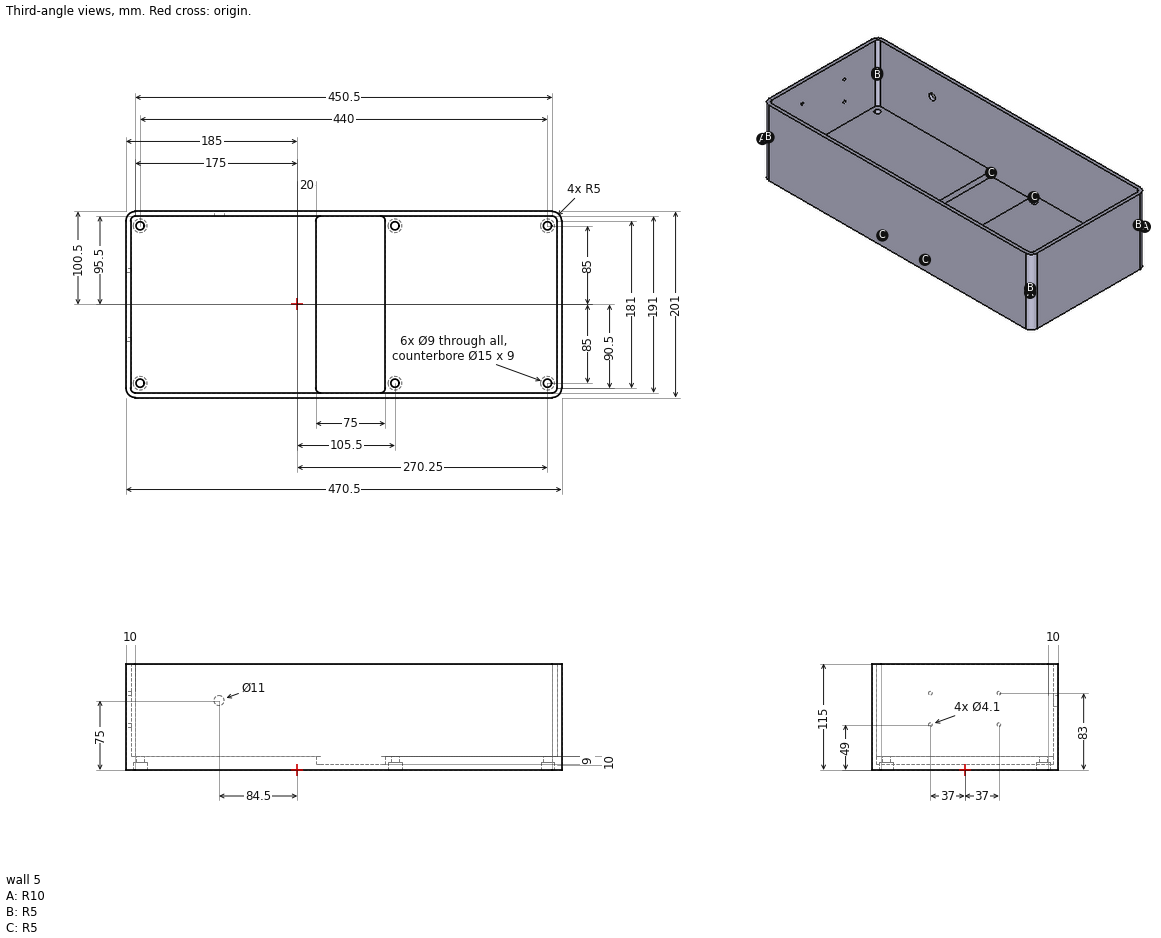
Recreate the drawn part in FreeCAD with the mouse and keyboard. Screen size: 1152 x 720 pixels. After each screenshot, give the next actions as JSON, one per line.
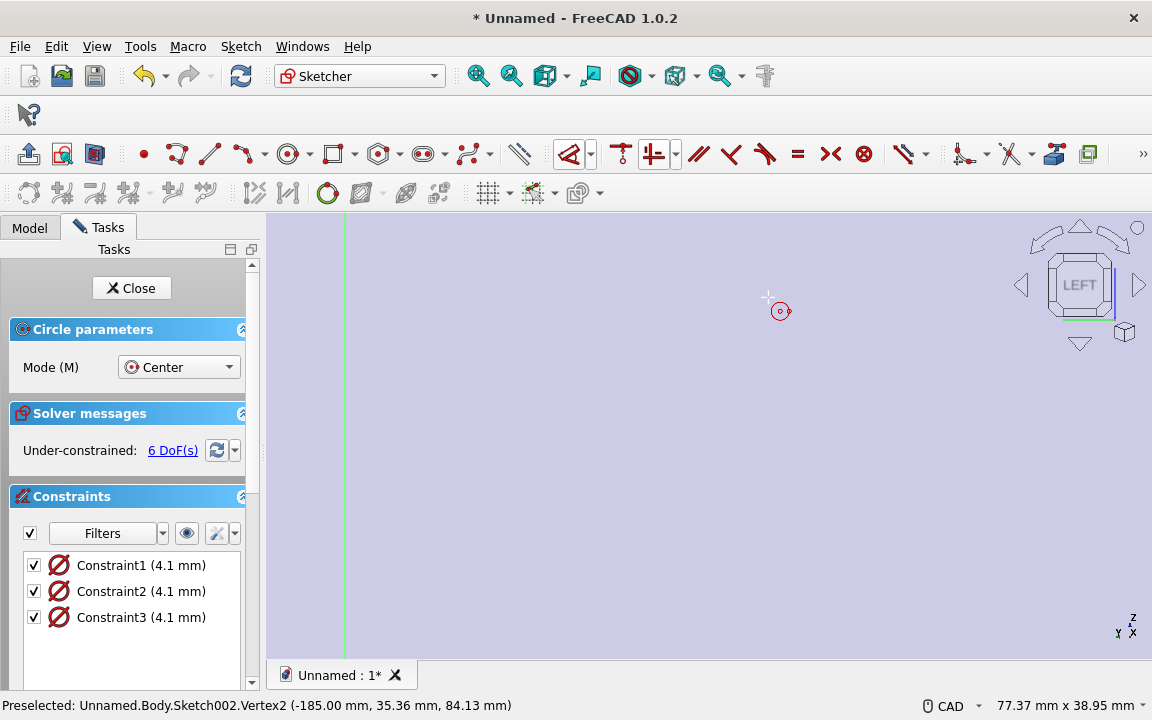
{"action": "left_click", "coordinate": [768, 295]}
{"action": "mouse_move", "coordinate": [785, 279]}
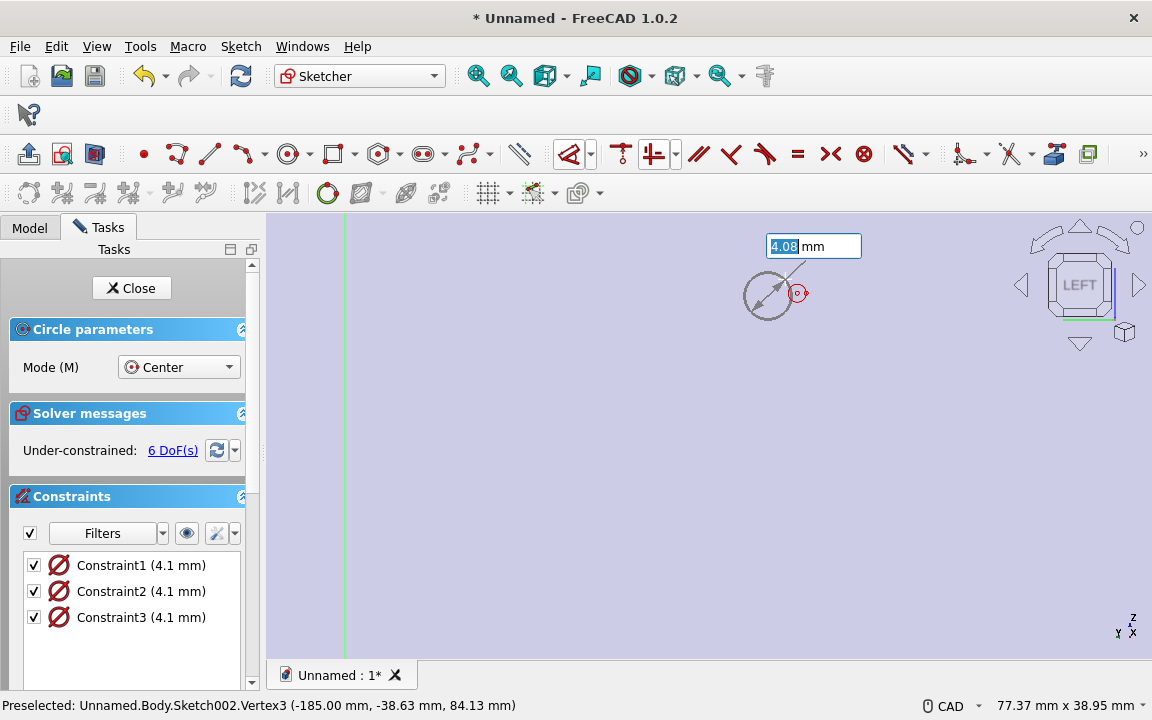
{"action": "type", "text": "4.1"}
{"action": "key", "text": "Return"}
{"action": "key", "text": "Escape"}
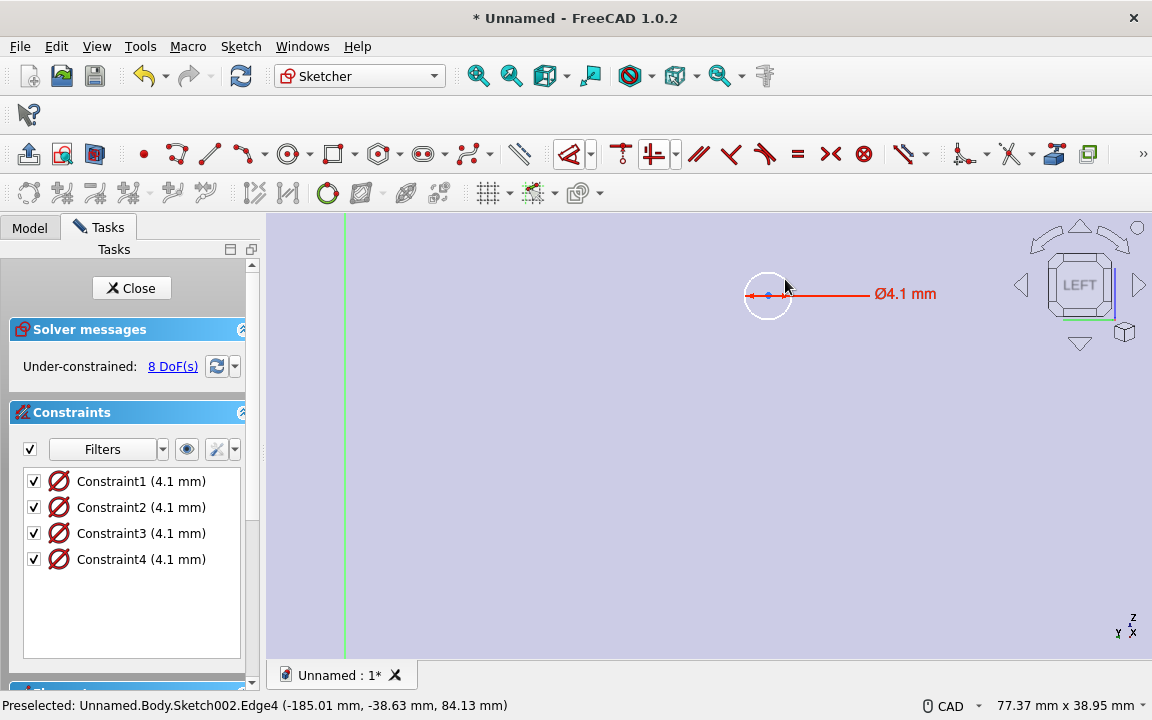
{"action": "scroll", "coordinate": [768, 297], "scroll_direction": "down", "scroll_amount": 6}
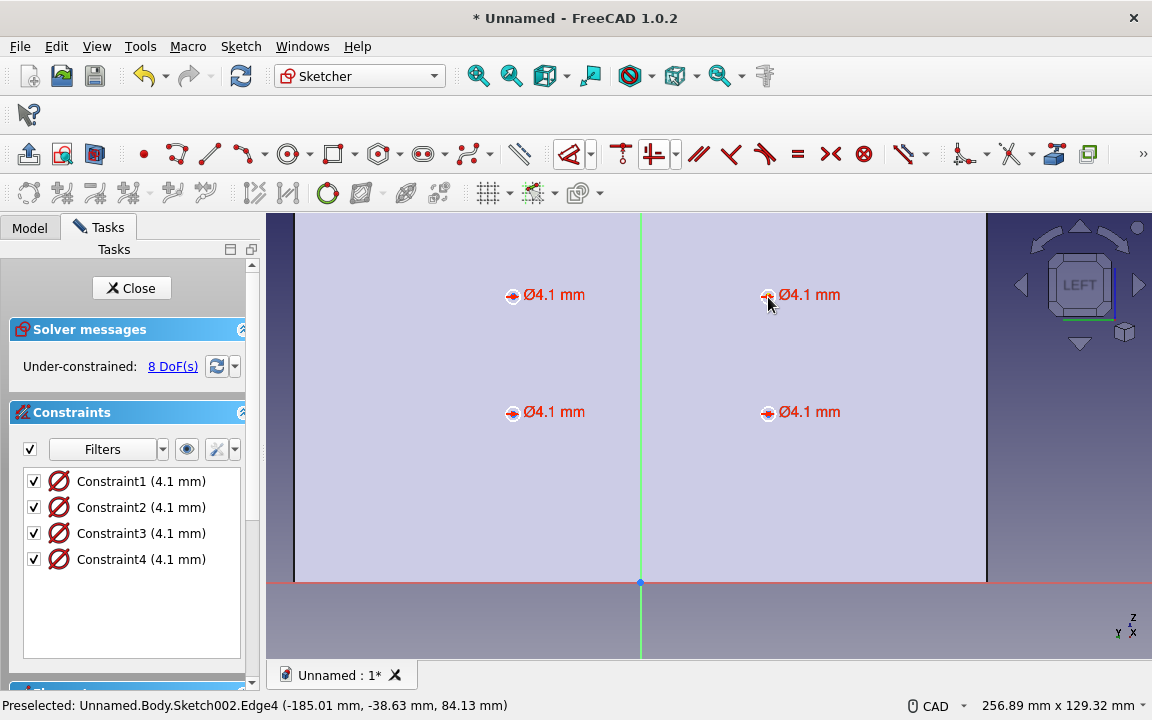
{"action": "left_click", "coordinate": [768, 414]}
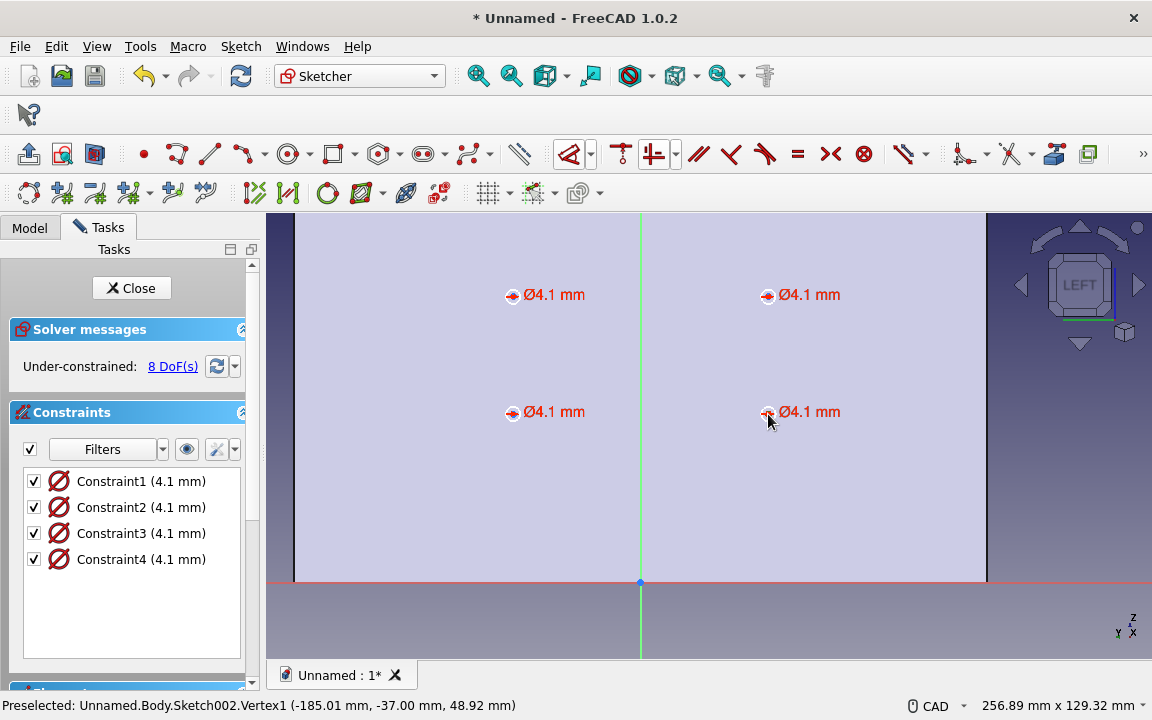
{"action": "left_click", "coordinate": [513, 414]}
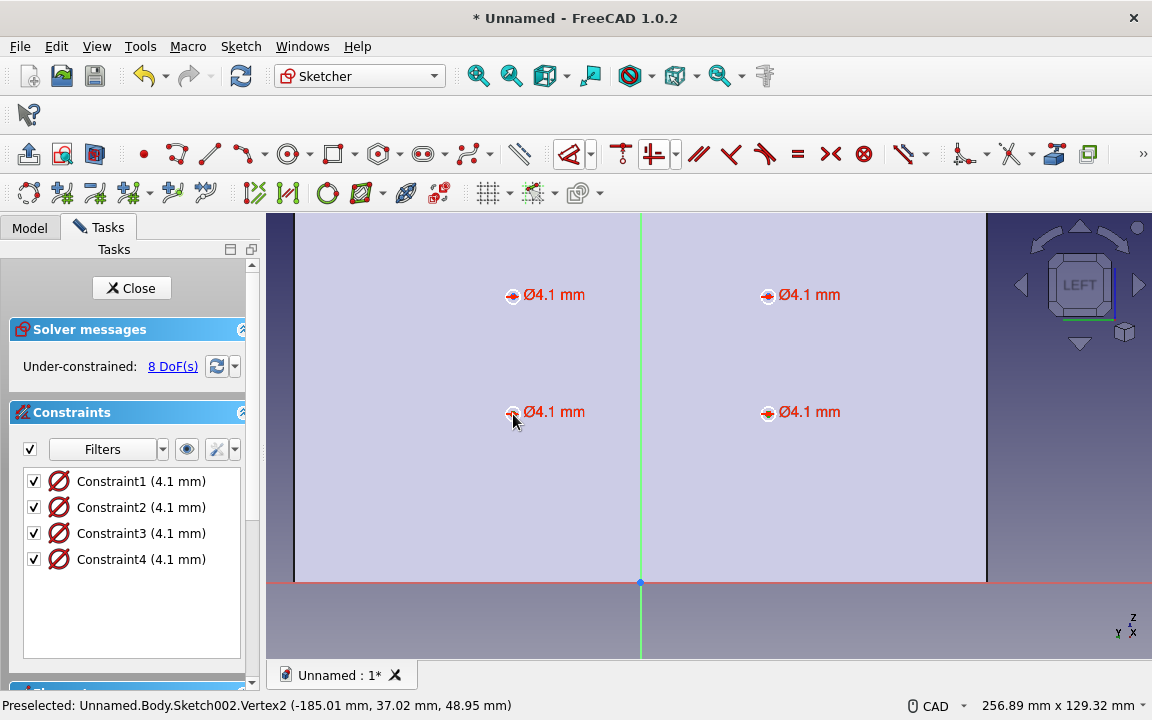
{"action": "key", "text": "h"}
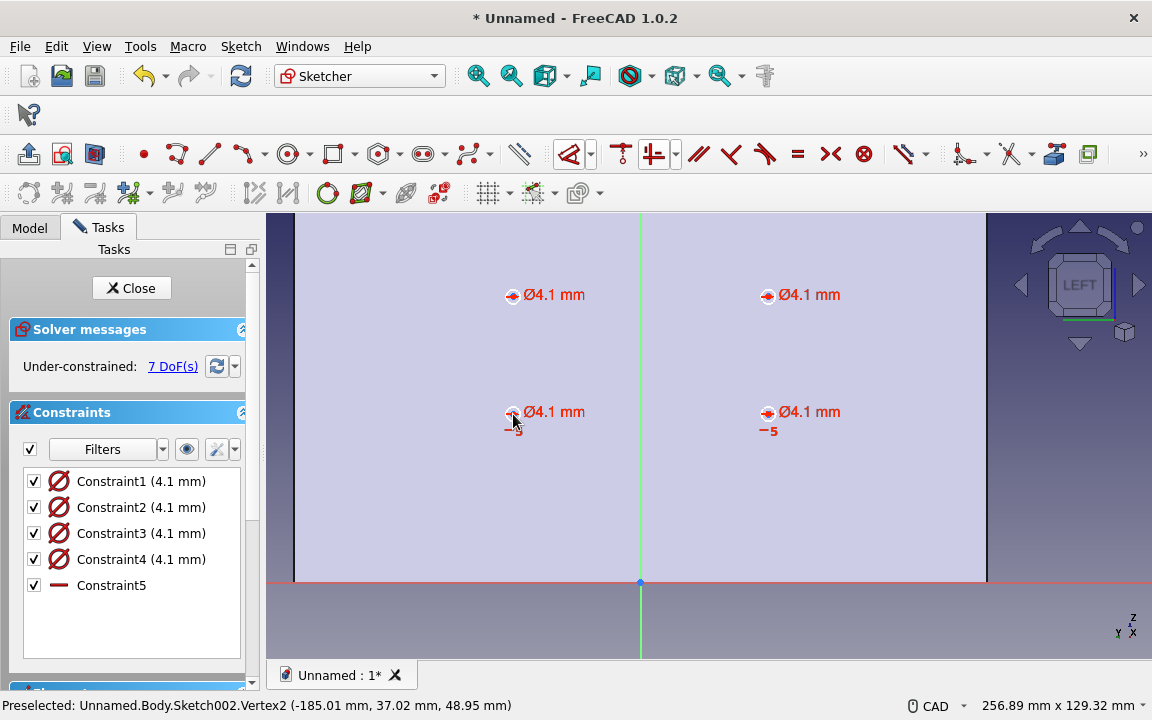
{"action": "left_click", "coordinate": [513, 414]}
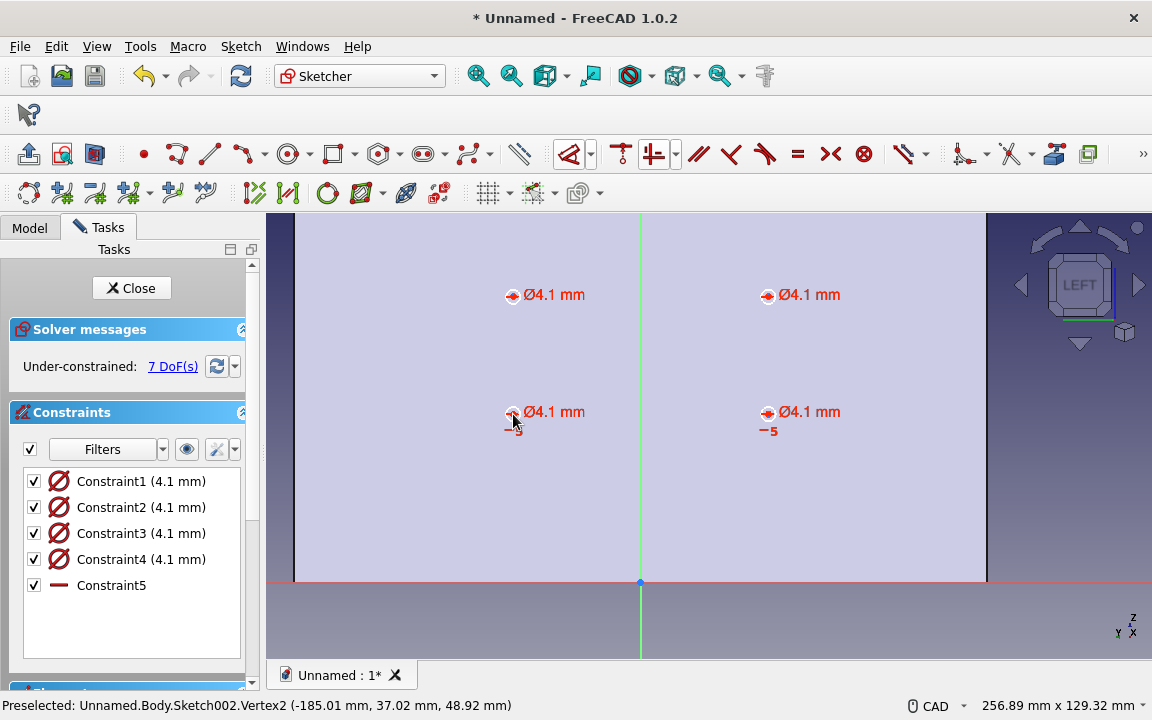
{"action": "left_click", "coordinate": [513, 297]}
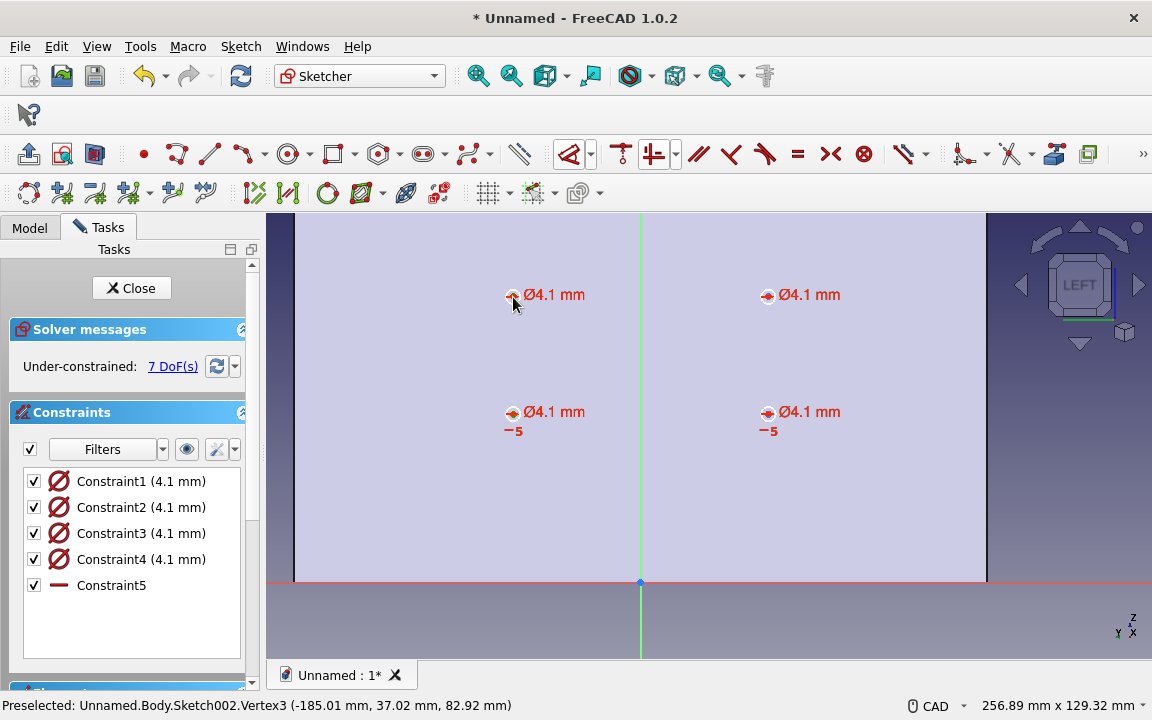
{"action": "key", "text": "v"}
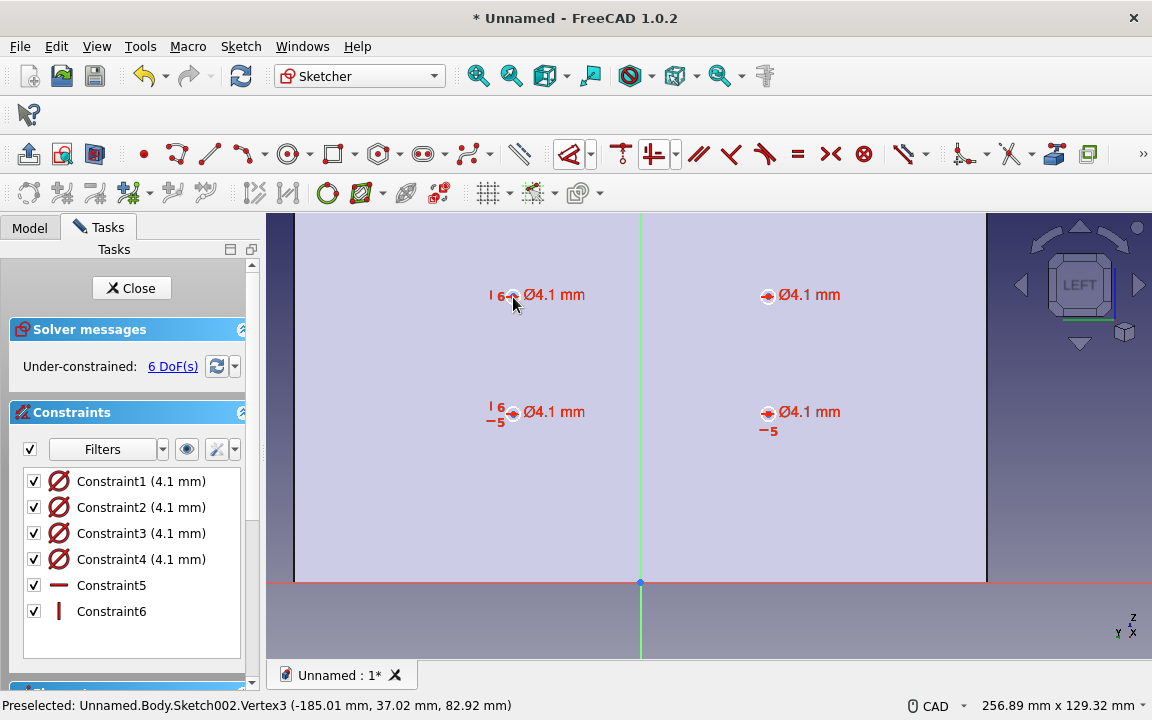
{"action": "left_click", "coordinate": [768, 414]}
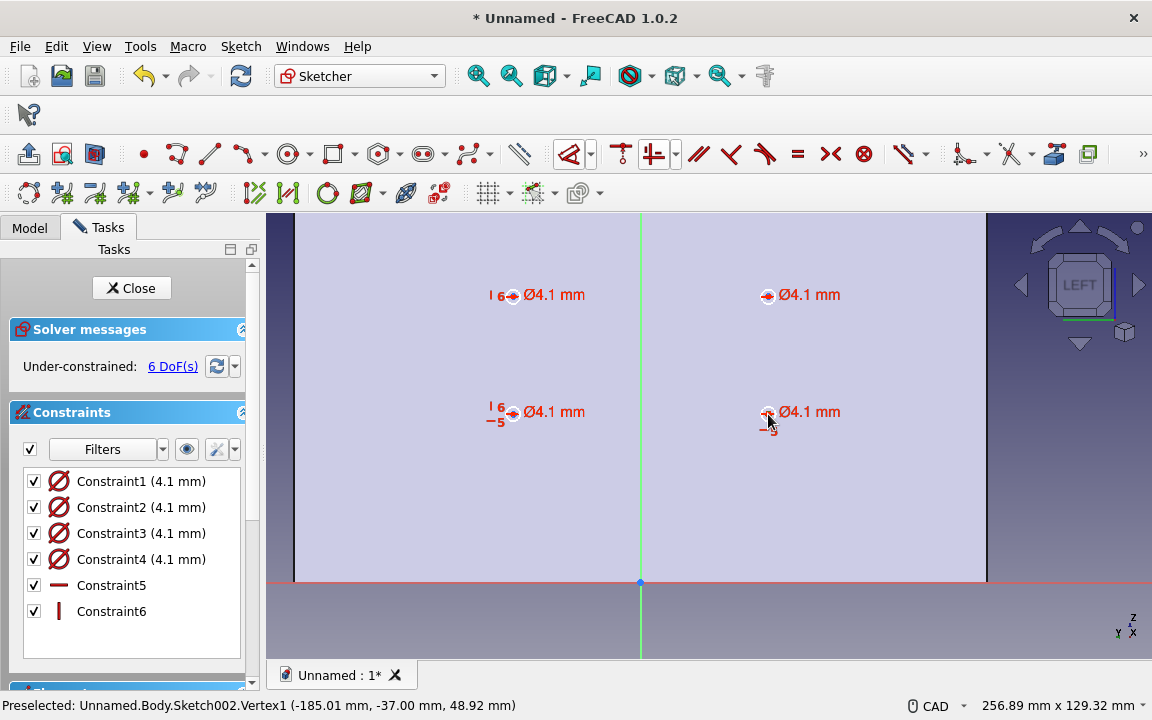
{"action": "left_click", "coordinate": [768, 297]}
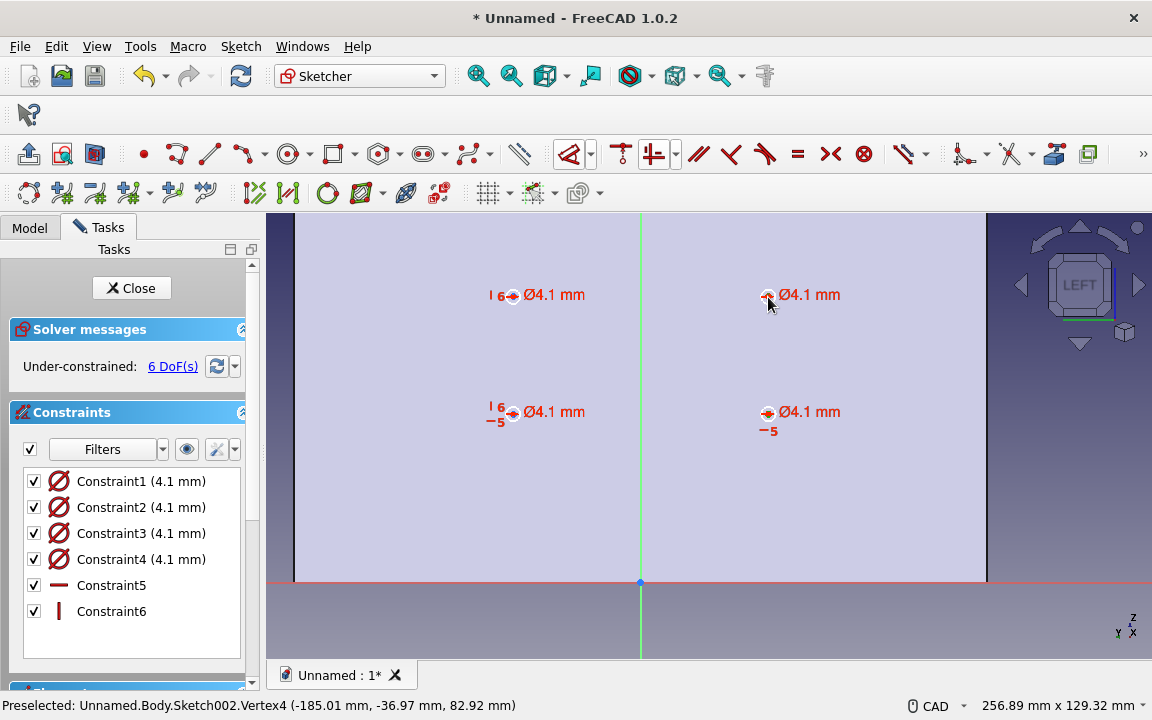
{"action": "key", "text": "v"}